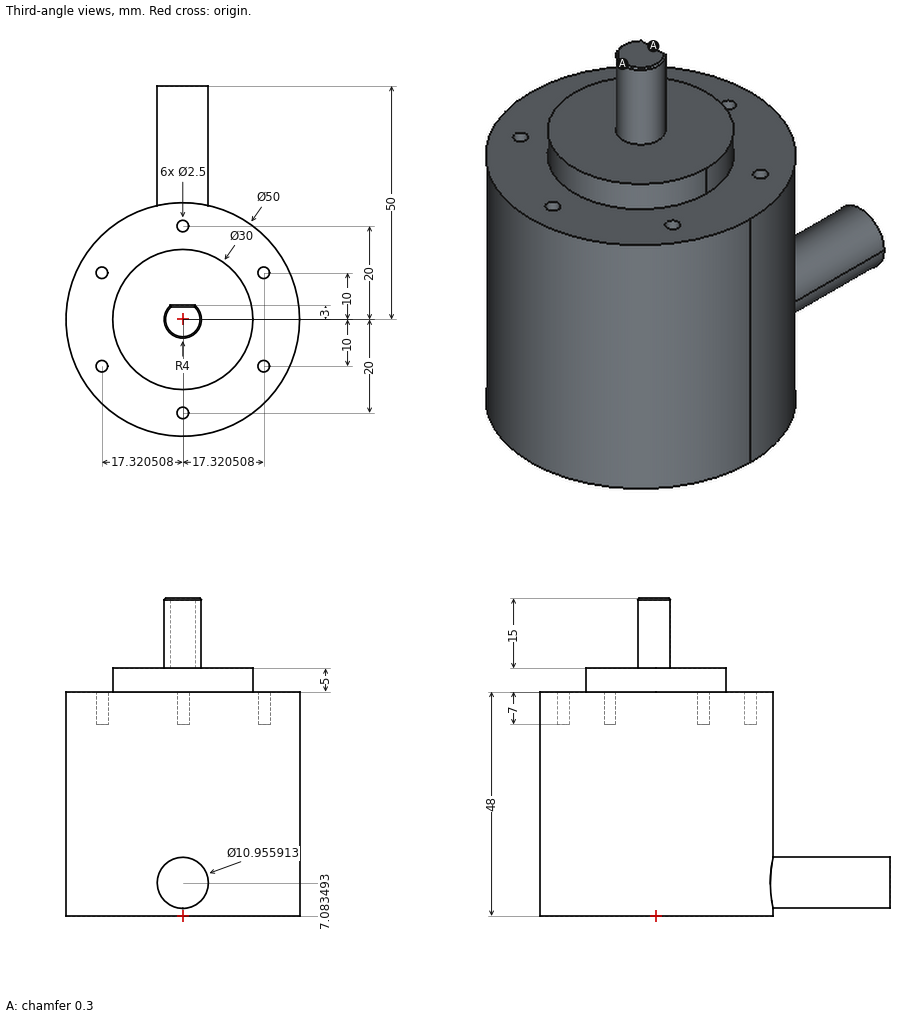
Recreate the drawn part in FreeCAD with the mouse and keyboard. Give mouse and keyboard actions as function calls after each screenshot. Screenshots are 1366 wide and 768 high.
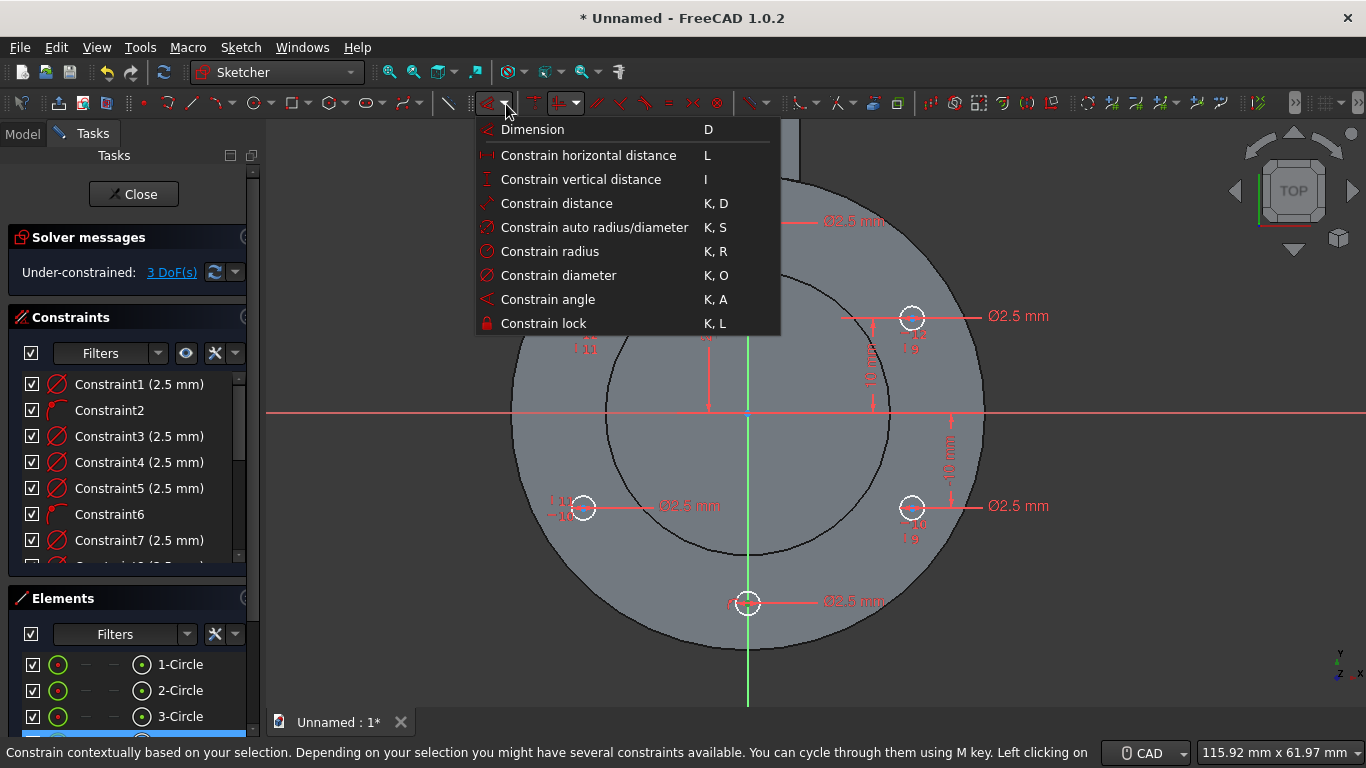
click(628, 179)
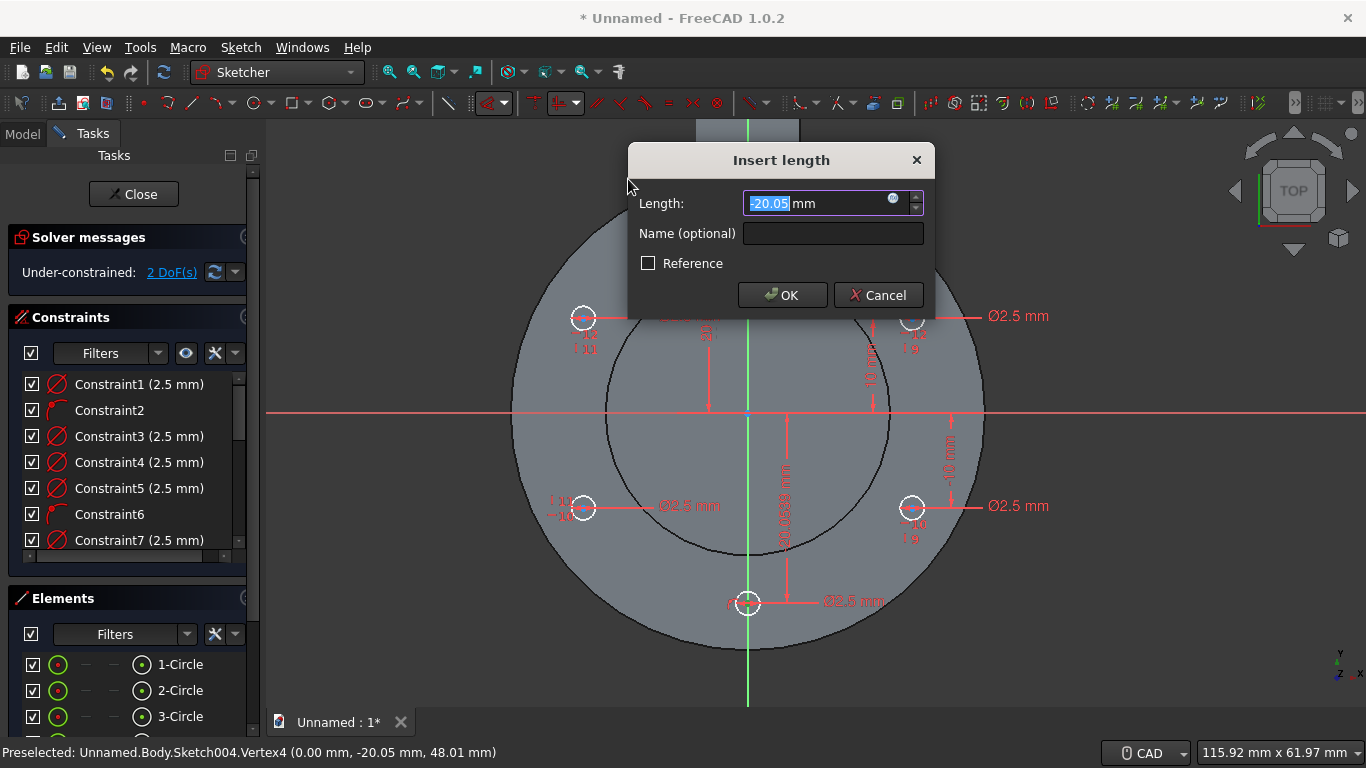
text(-20)
key(Return)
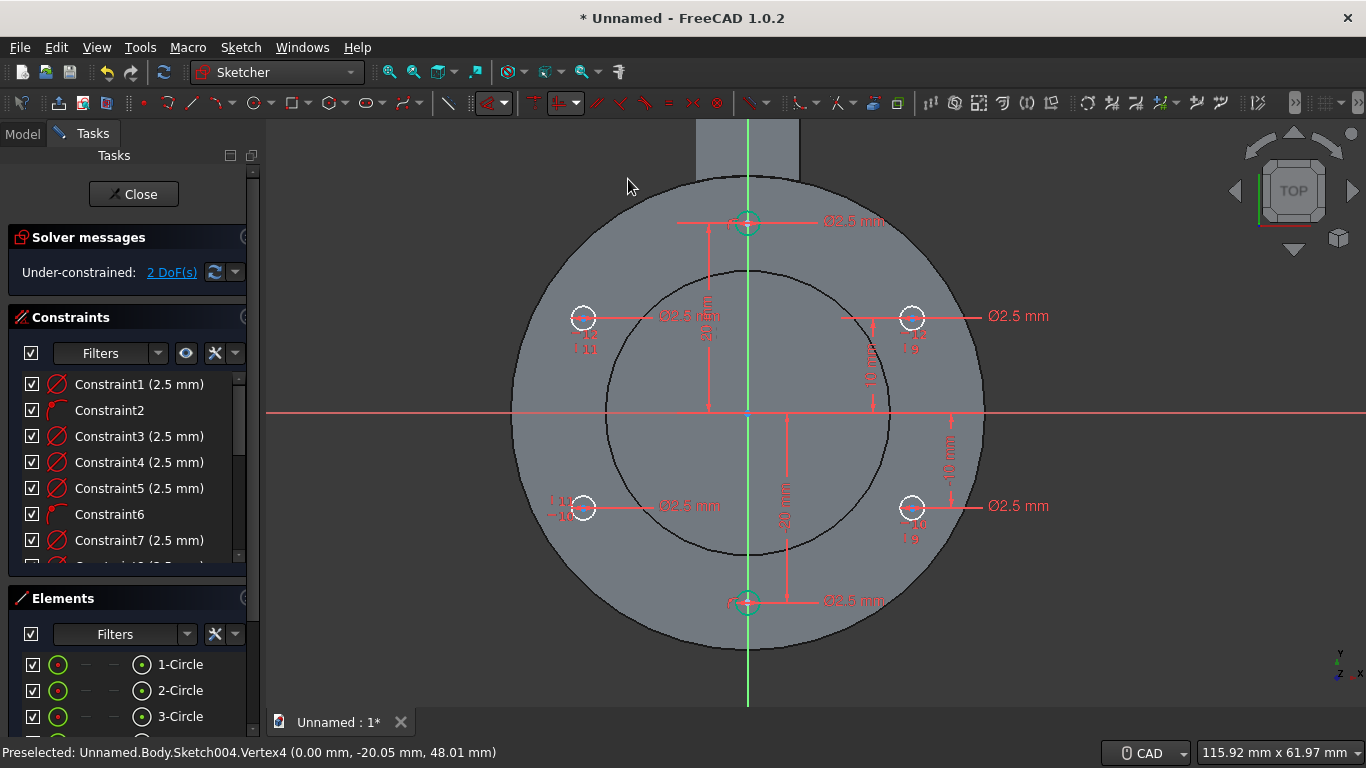
click(912, 318)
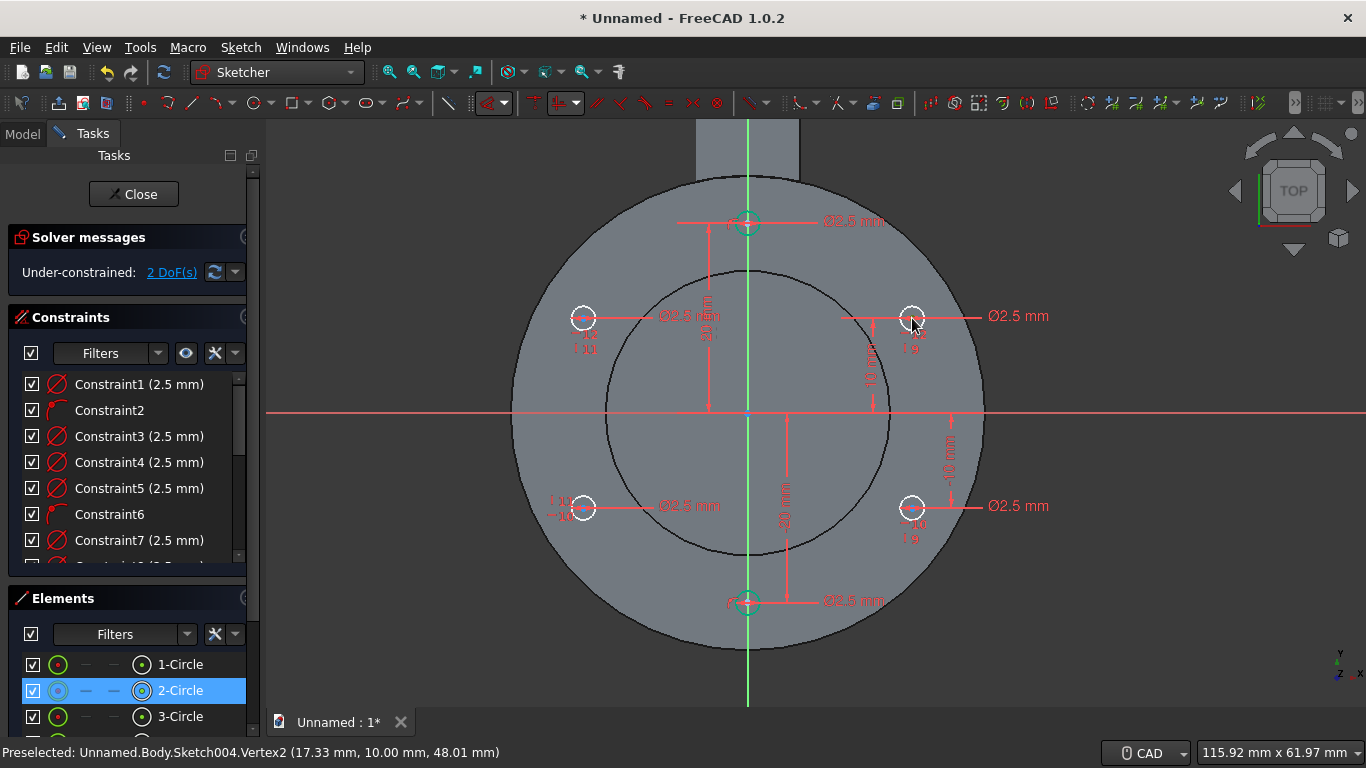
click(506, 104)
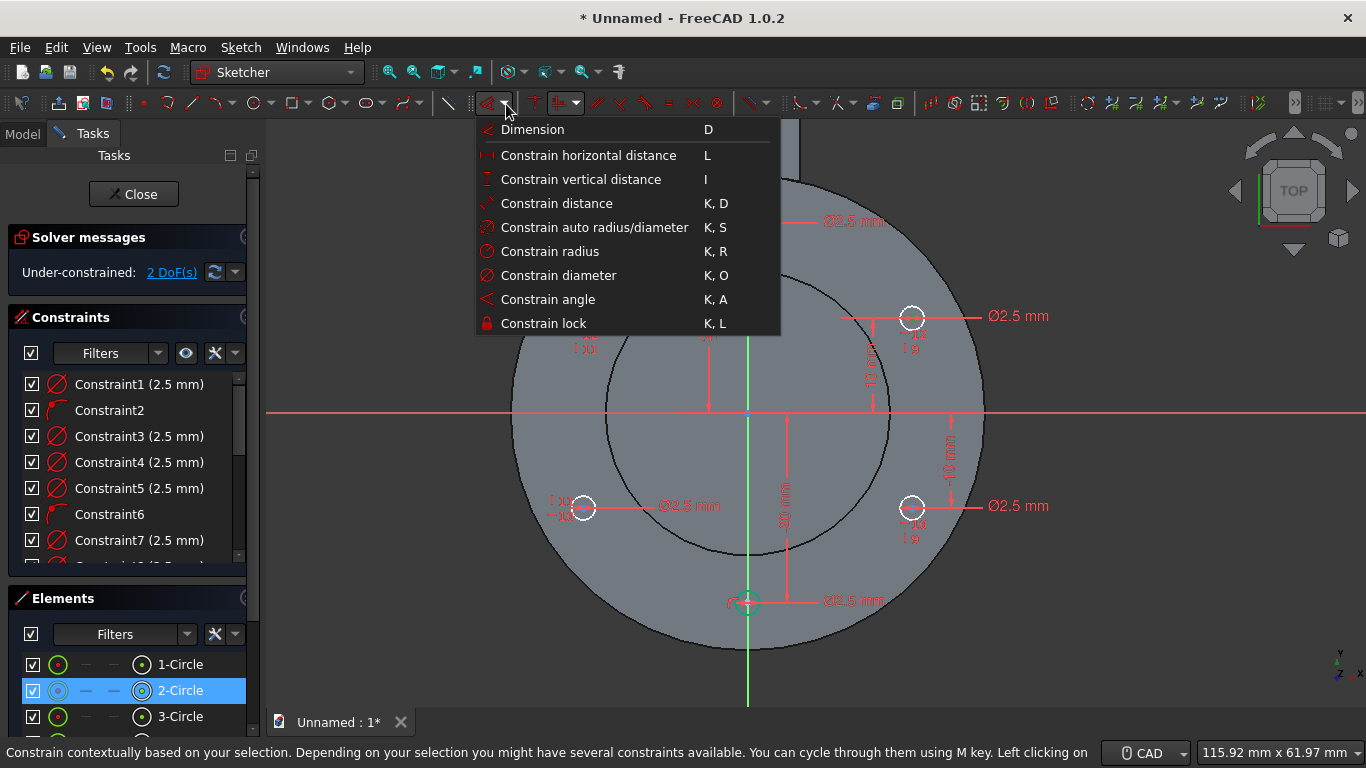
click(628, 155)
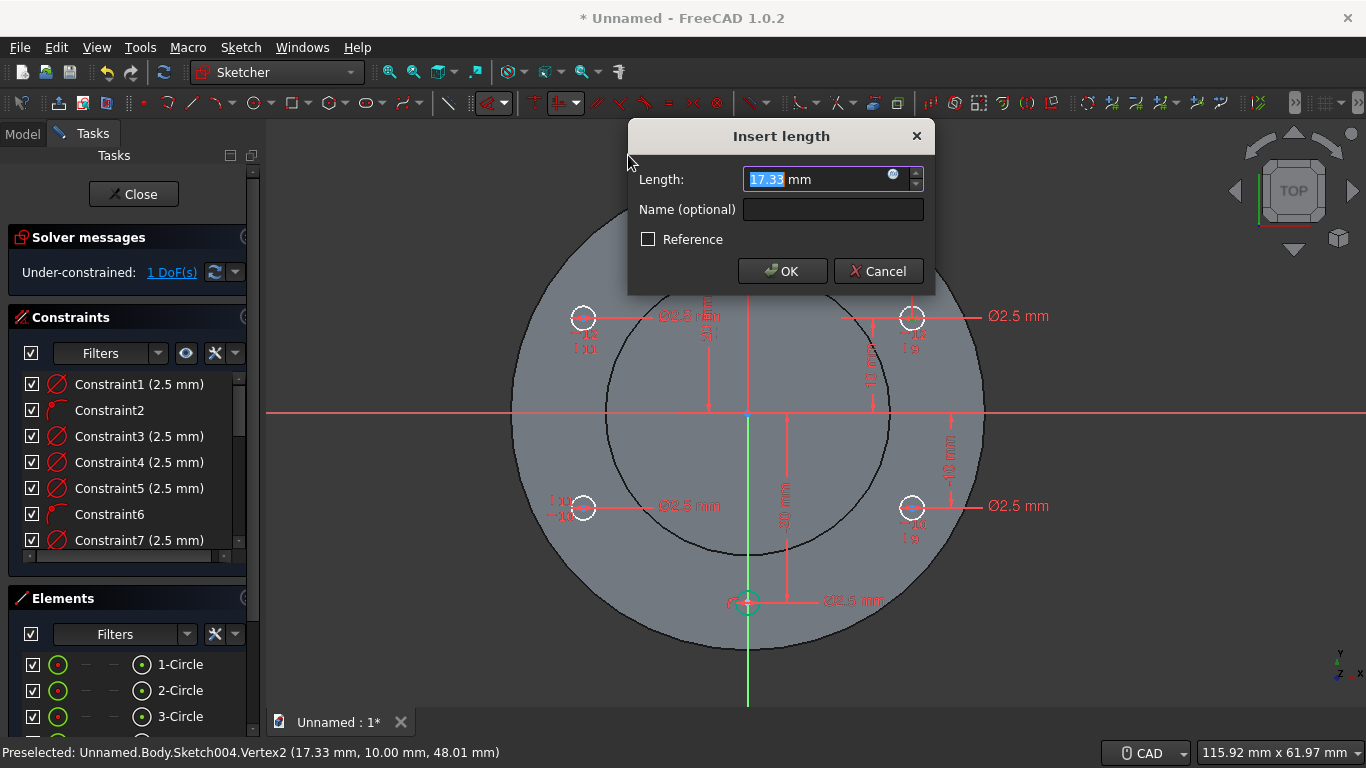
text(17.320508)
key(Return)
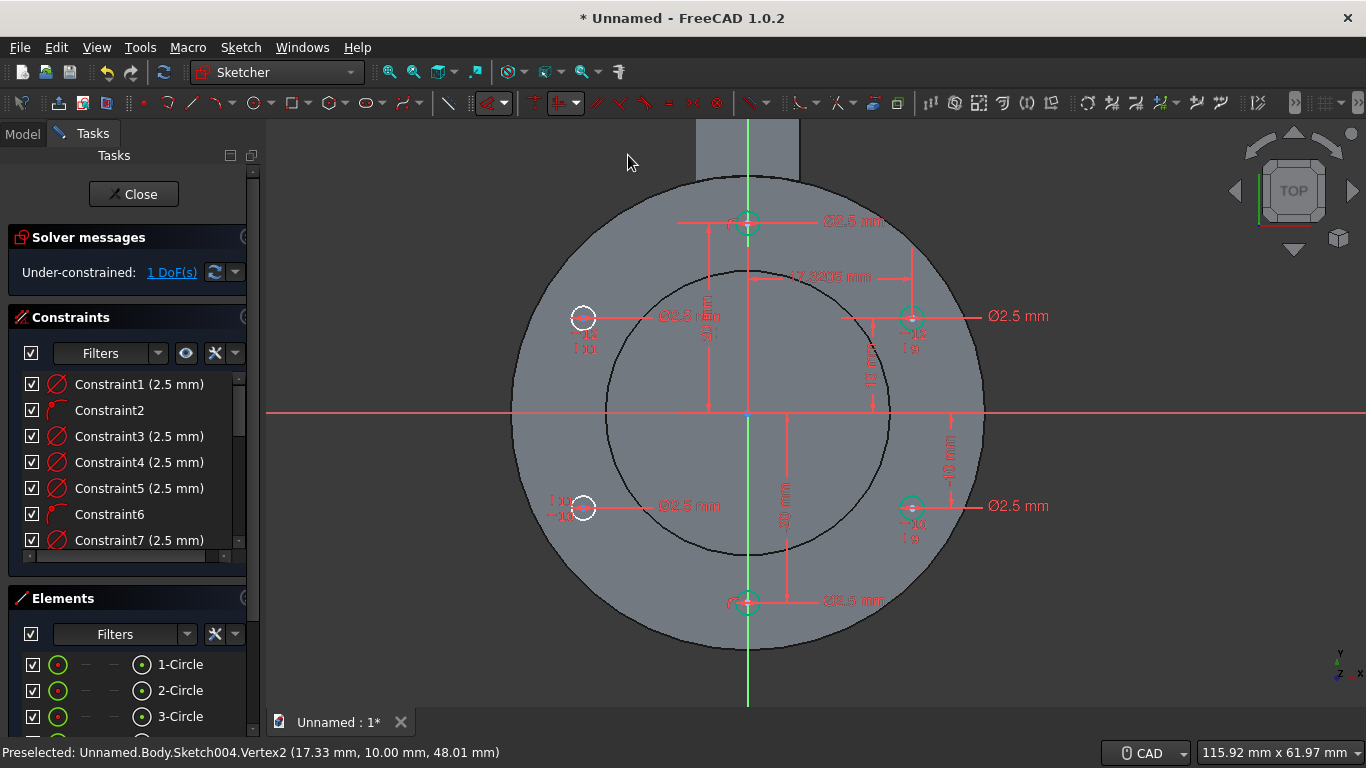
click(583, 508)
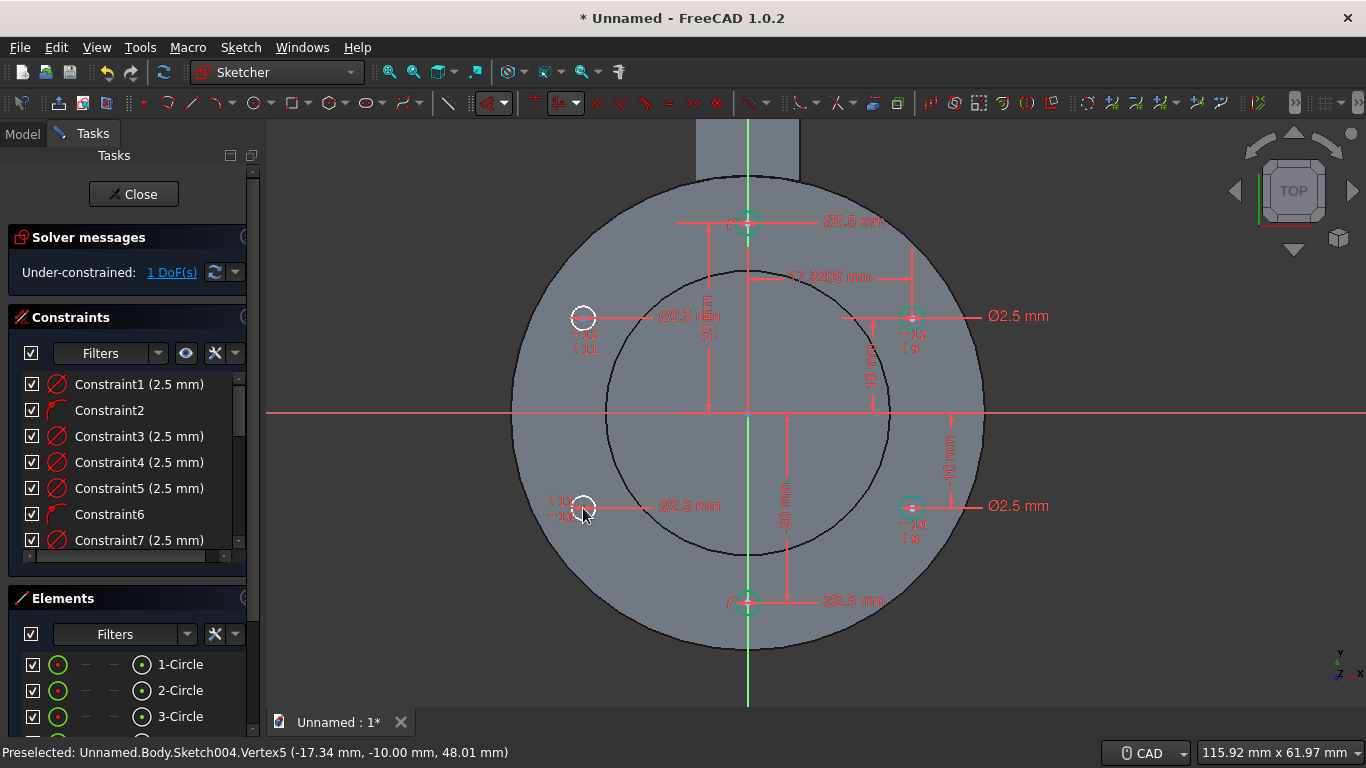
key(l)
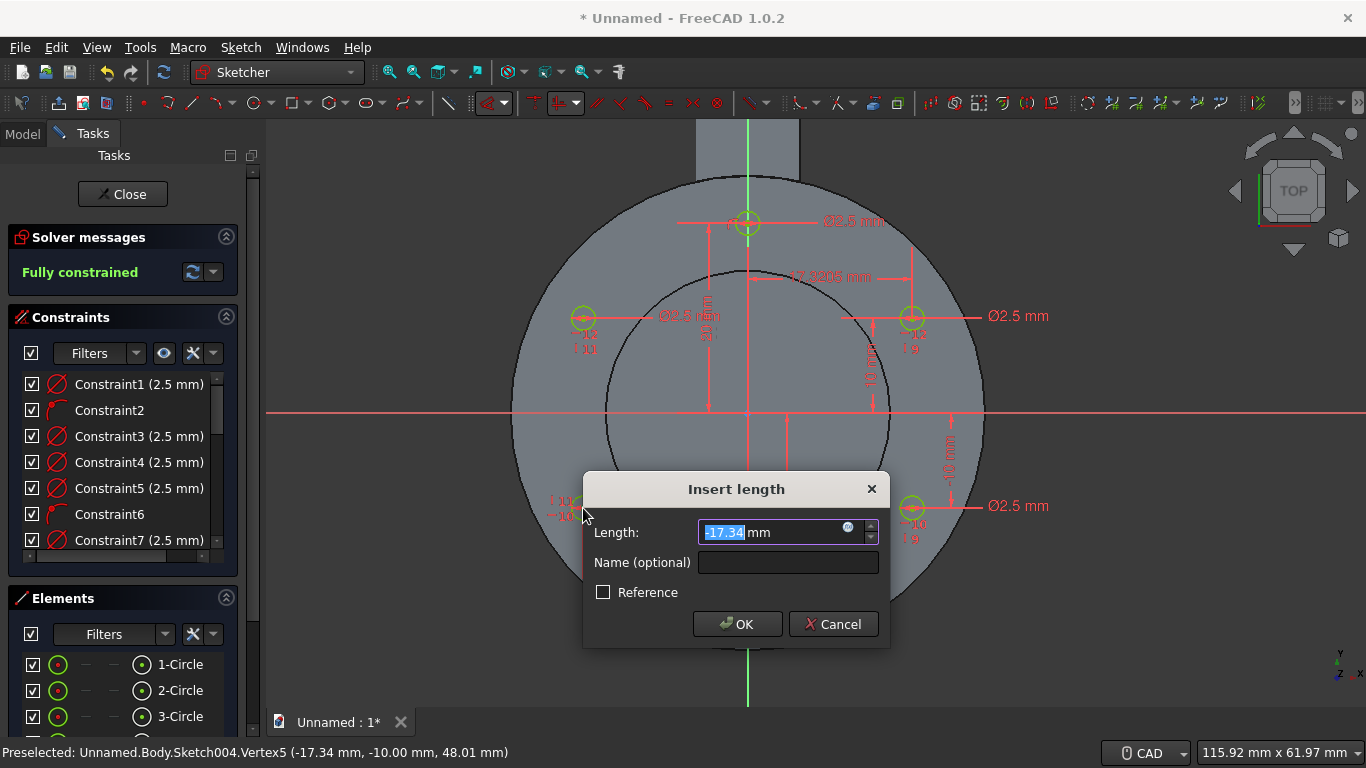
text(-17.320508)
key(Return)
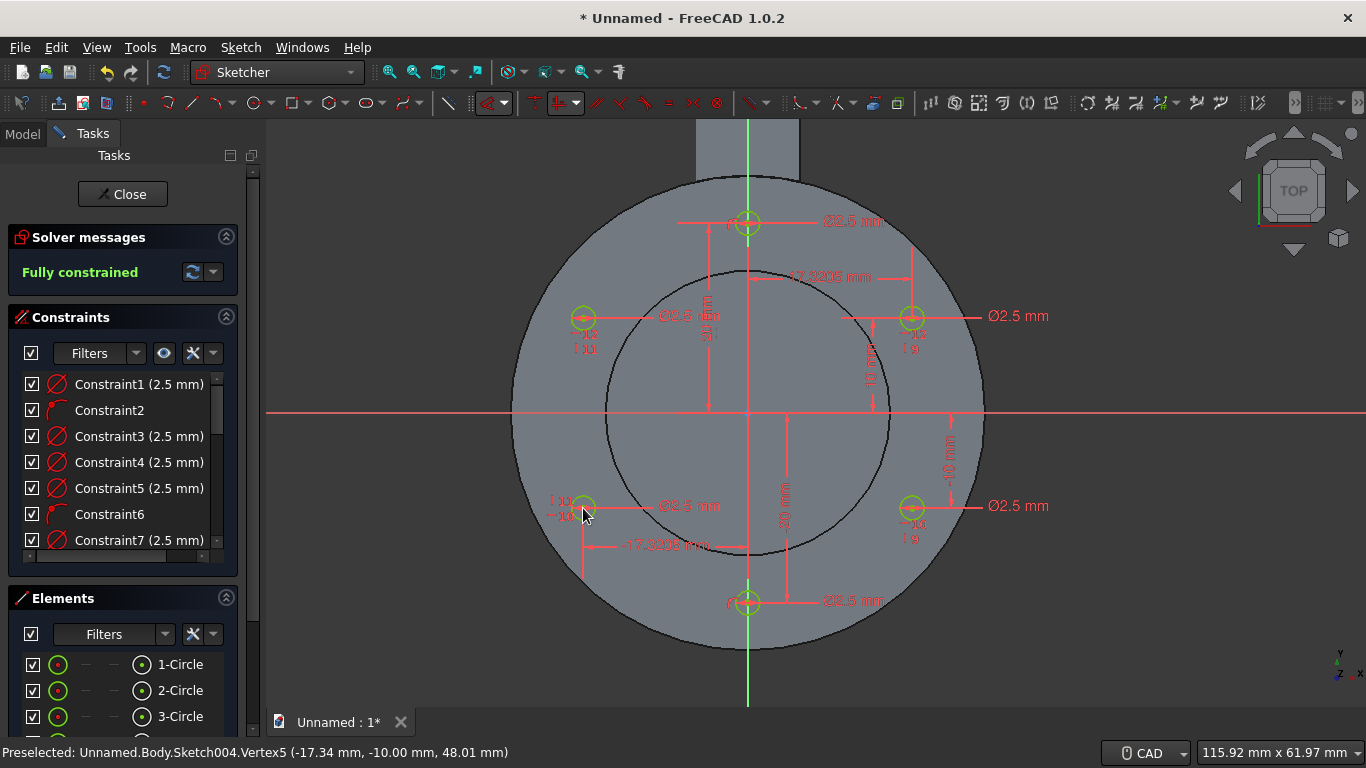
click(123, 194)